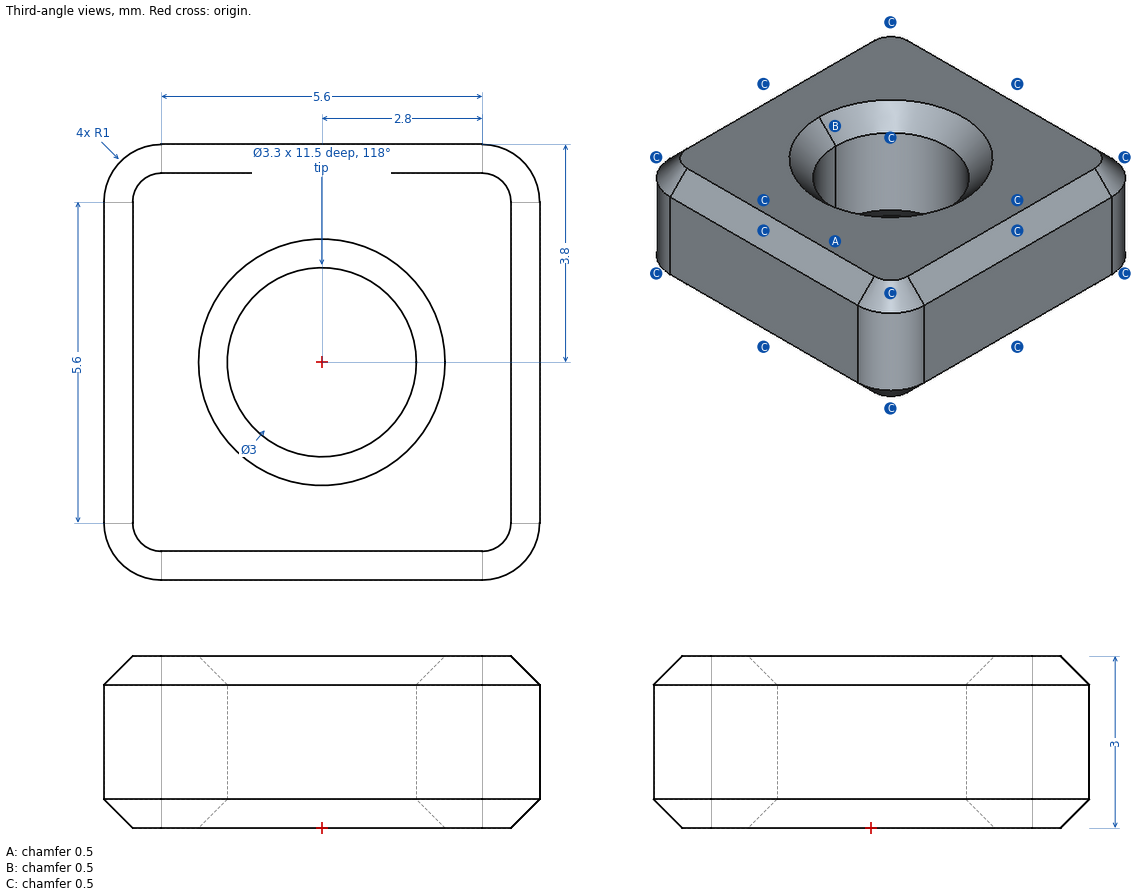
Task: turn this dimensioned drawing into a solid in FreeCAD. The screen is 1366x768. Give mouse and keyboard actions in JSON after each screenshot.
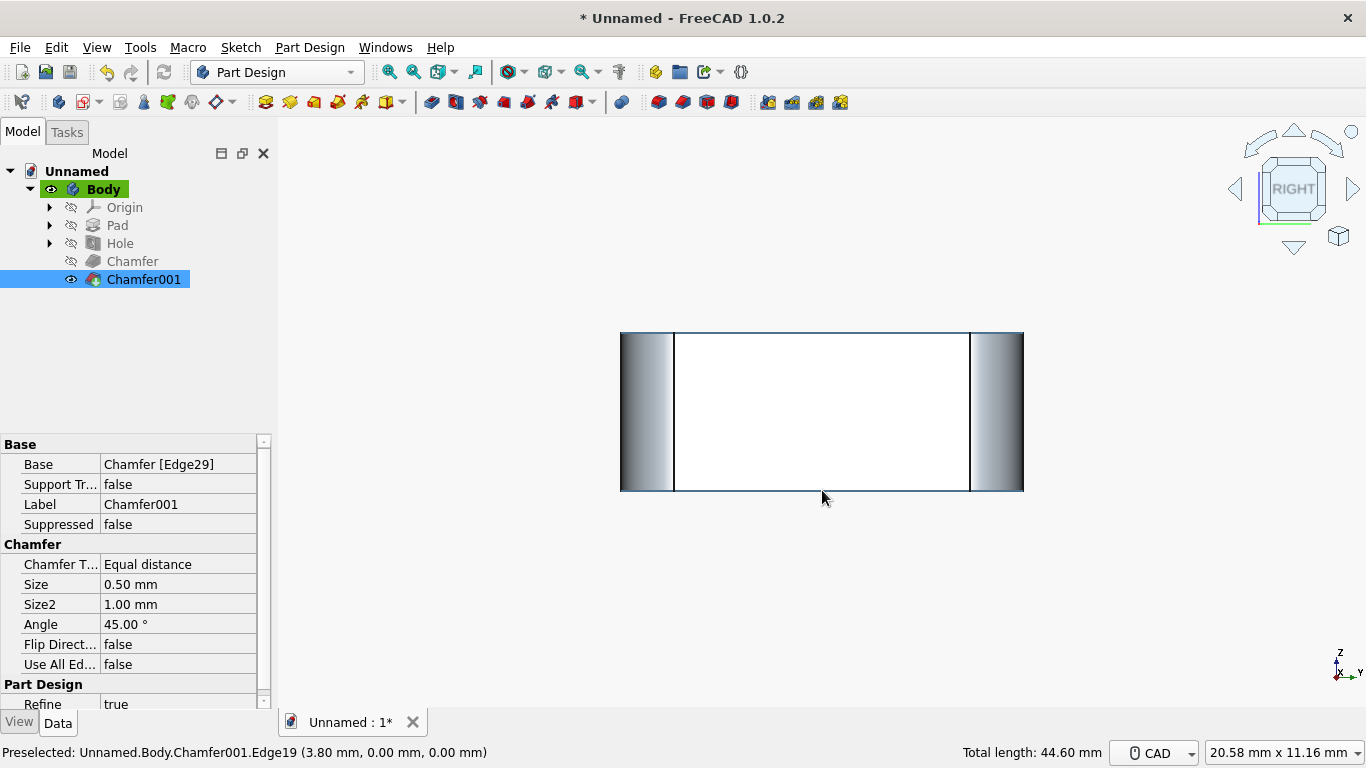
{"action": "key", "text": "5"}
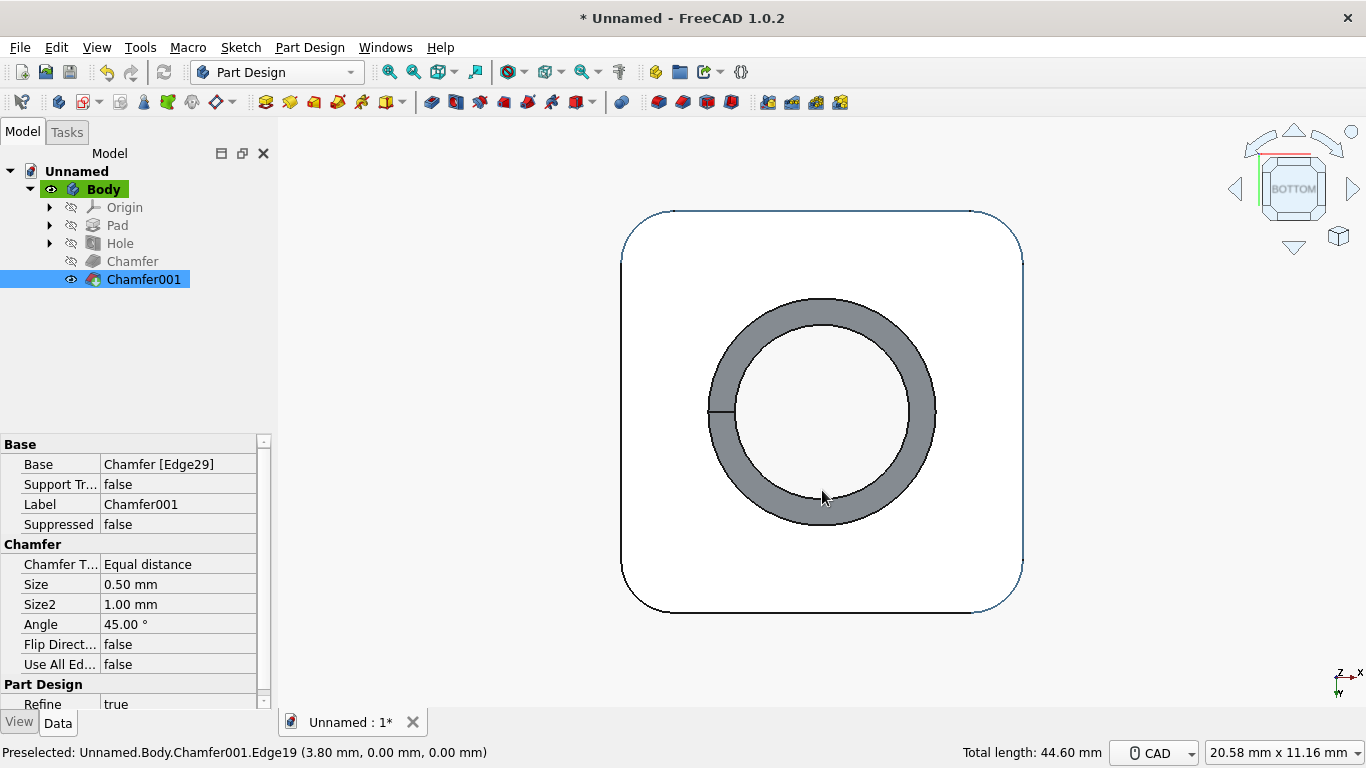
{"action": "left_click", "coordinate": [621, 411], "text": "ctrl"}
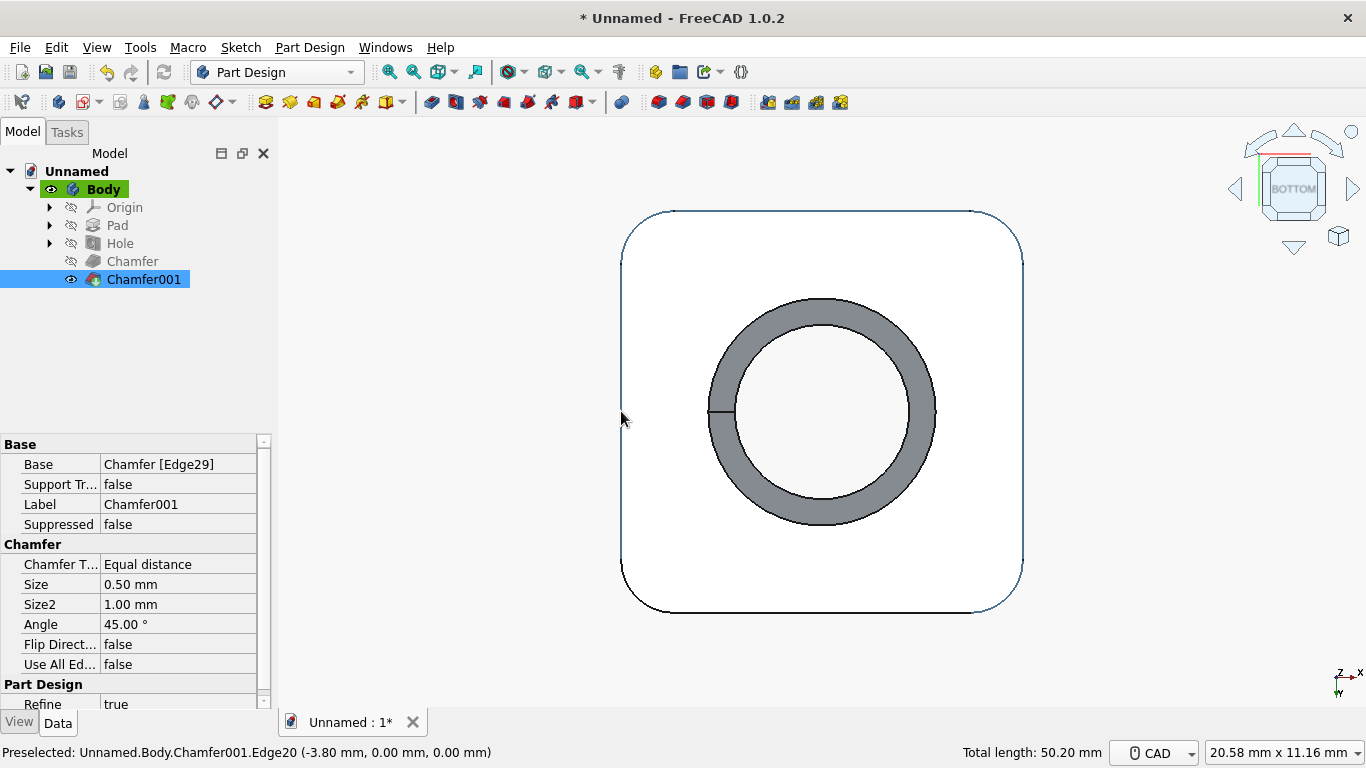
{"action": "left_click", "coordinate": [637, 596], "text": "ctrl"}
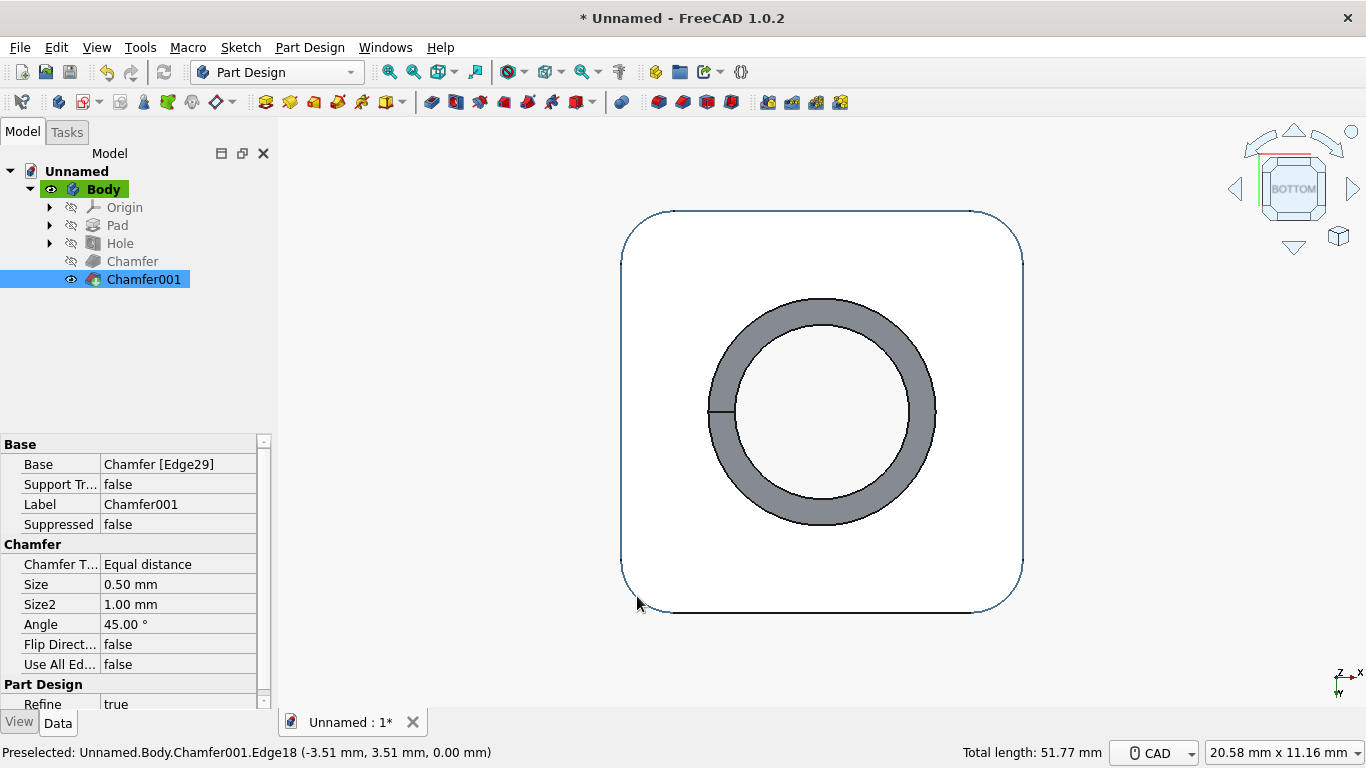
{"action": "left_click", "coordinate": [822, 612], "text": "ctrl"}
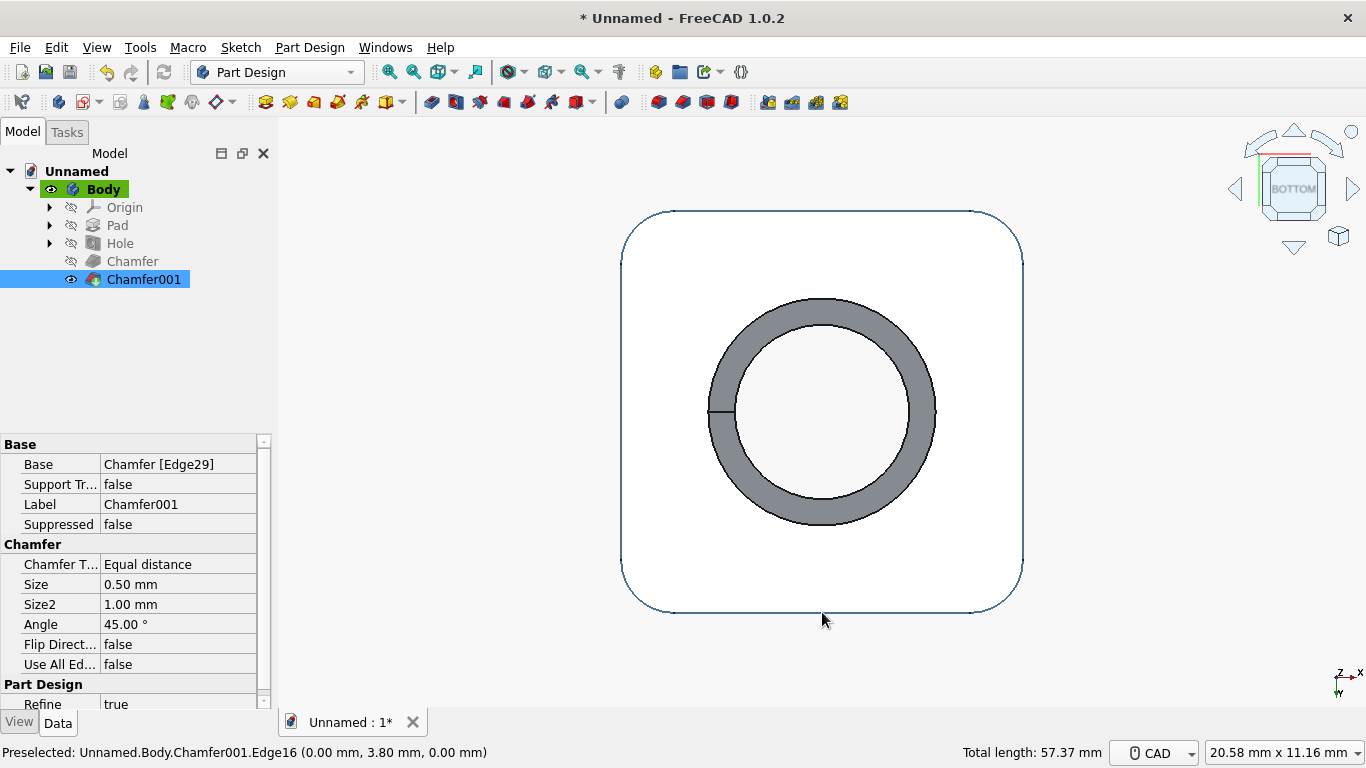
{"action": "left_click", "coordinate": [684, 102]}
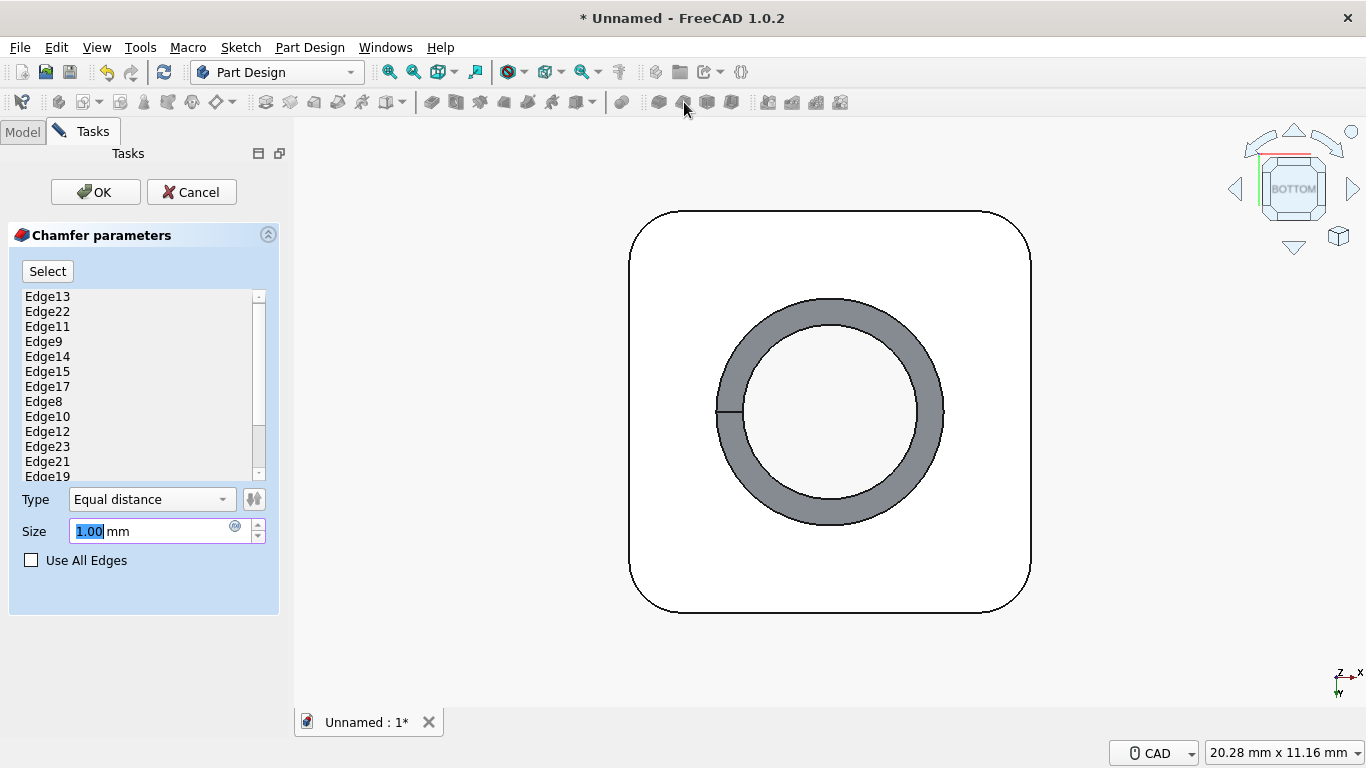
{"action": "type", "text": "0.5"}
{"action": "key", "text": "Tab"}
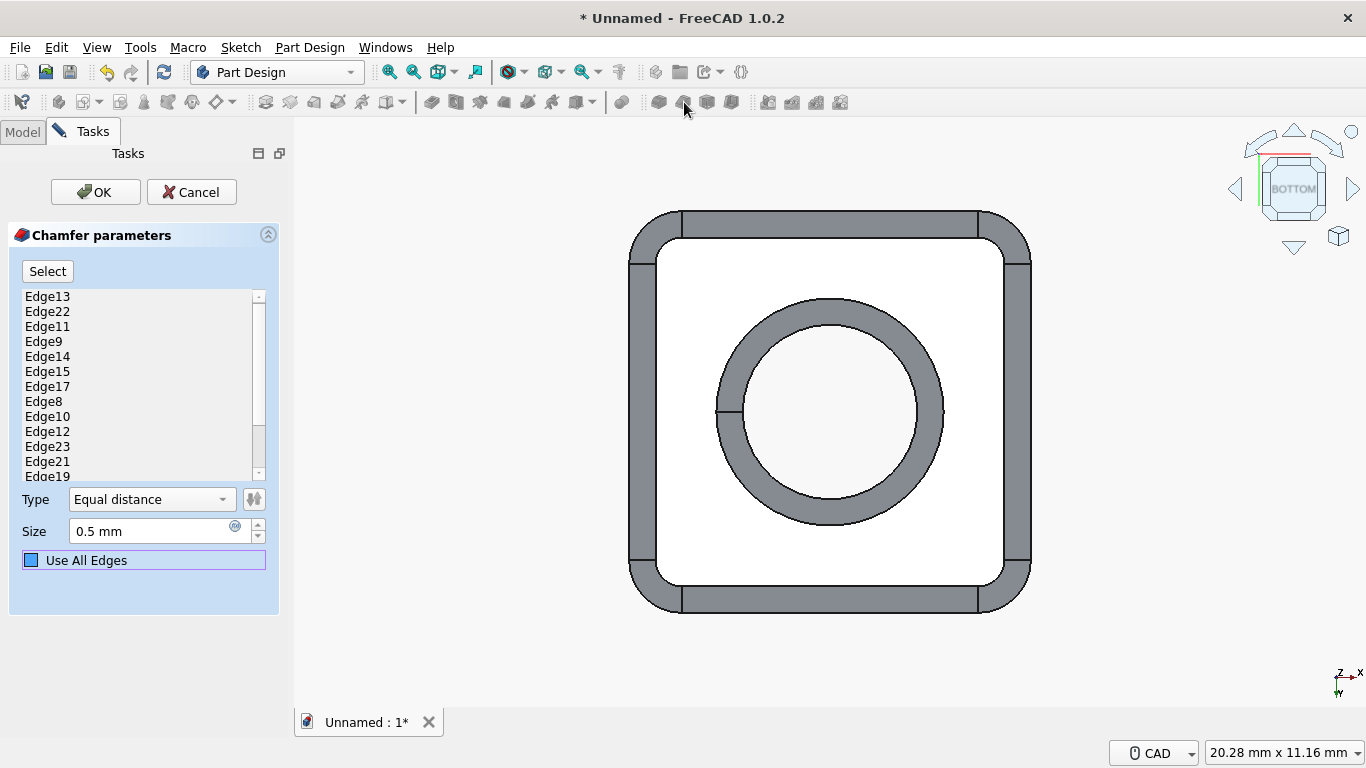
{"action": "left_click", "coordinate": [96, 192]}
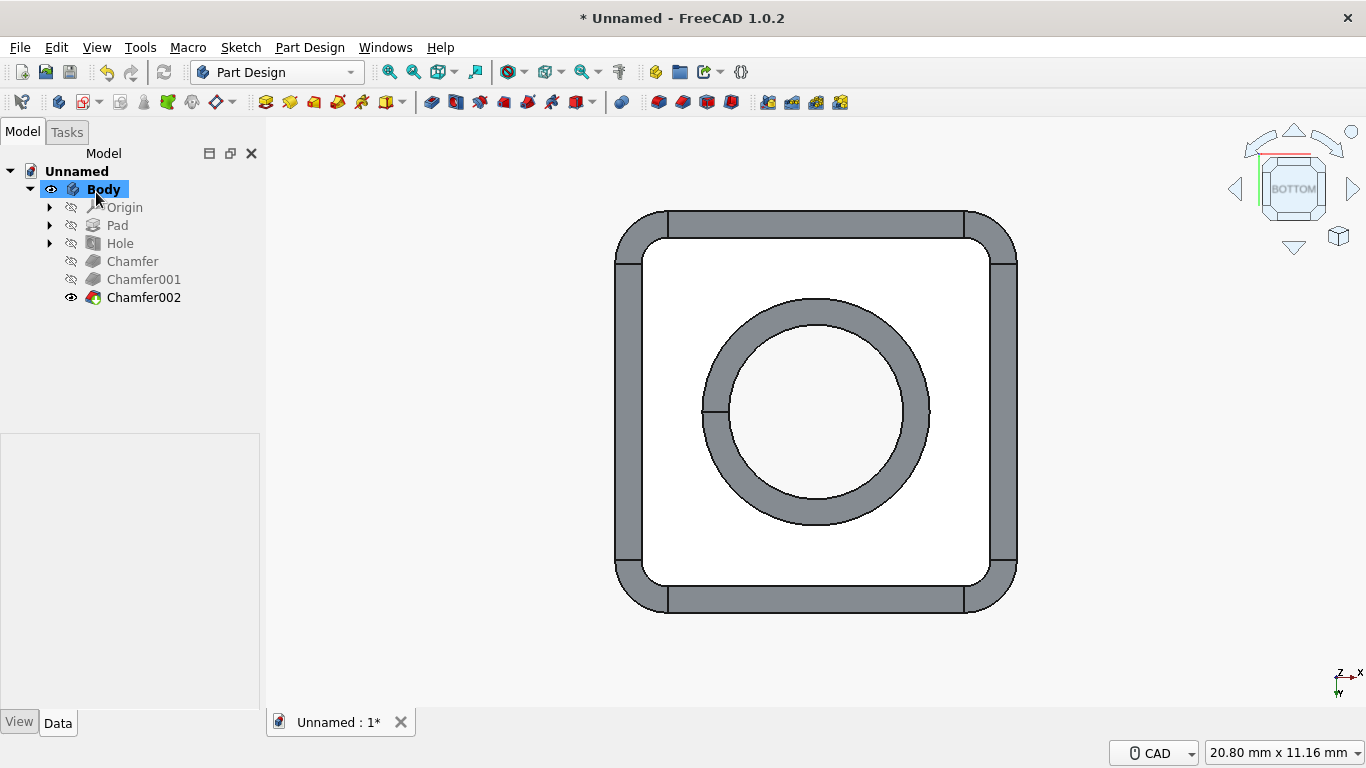
{"action": "key", "text": "0"}